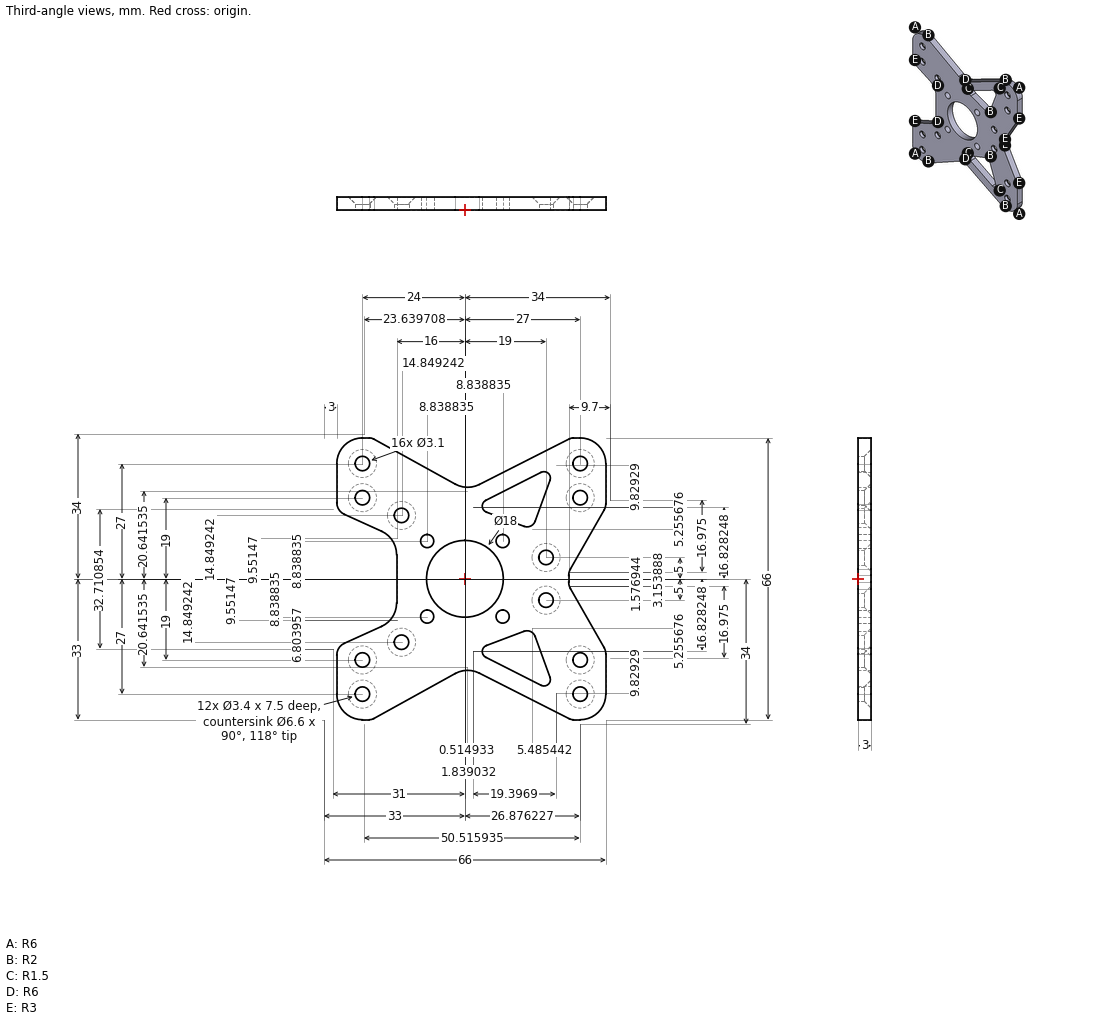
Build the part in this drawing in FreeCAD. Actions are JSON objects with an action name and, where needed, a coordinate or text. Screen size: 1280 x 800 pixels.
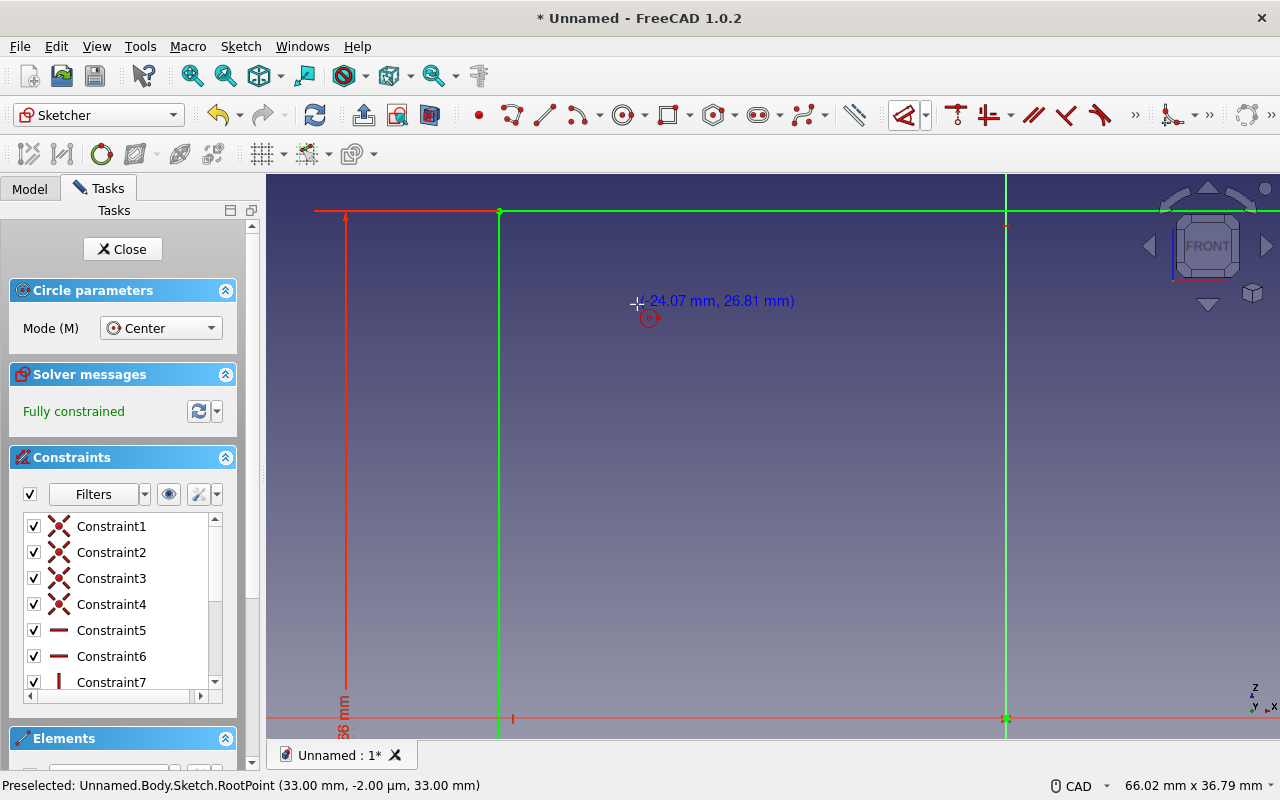
{"action": "left_click", "coordinate": [637, 303]}
{"action": "mouse_move", "coordinate": [654, 287]}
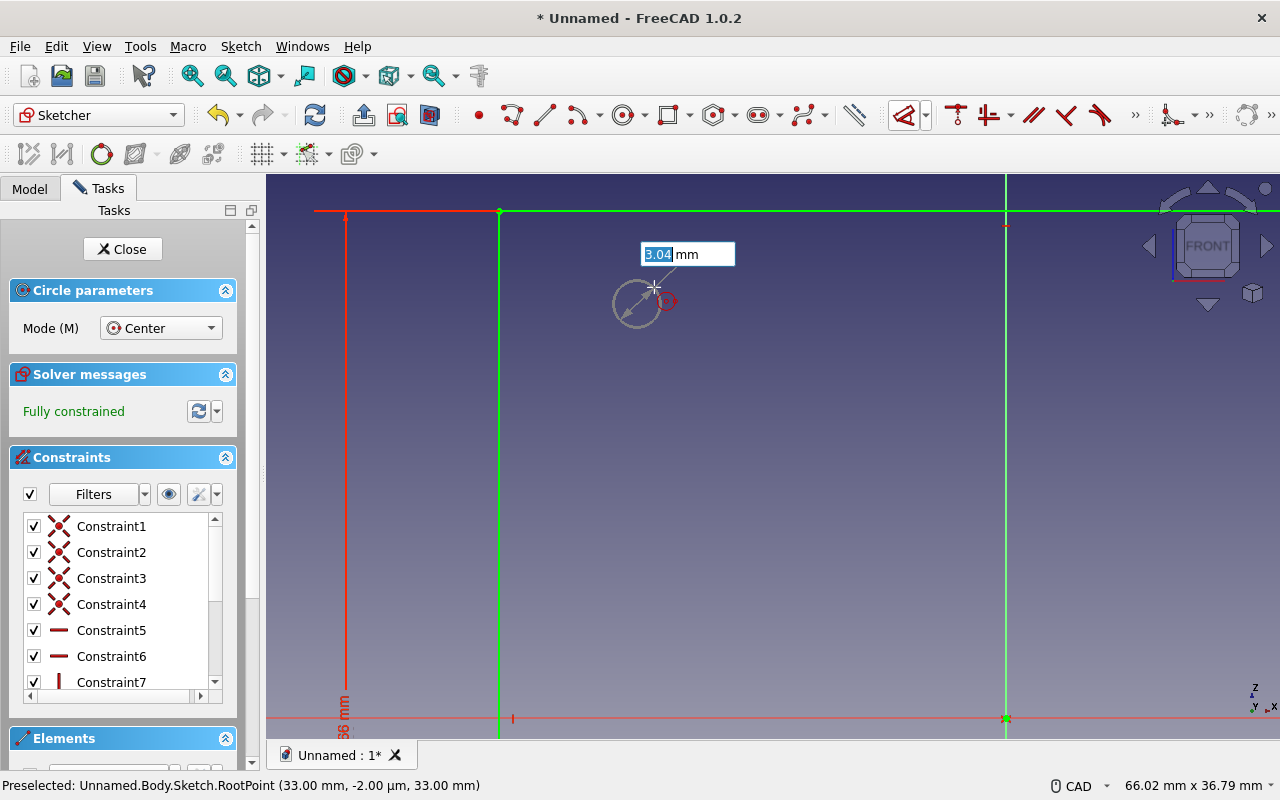
{"action": "type", "text": "3.1"}
{"action": "key", "text": "Return"}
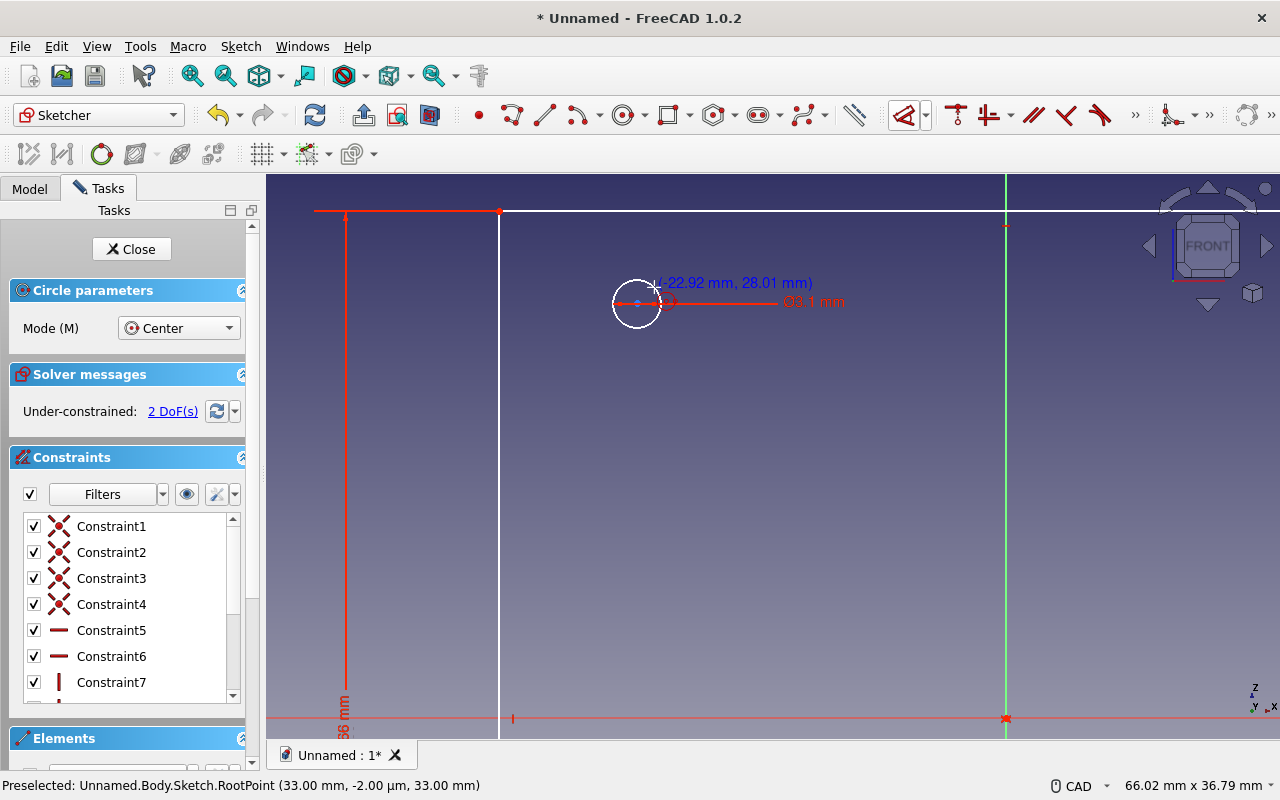
{"action": "left_click", "coordinate": [637, 426]}
{"action": "mouse_move", "coordinate": [654, 410]}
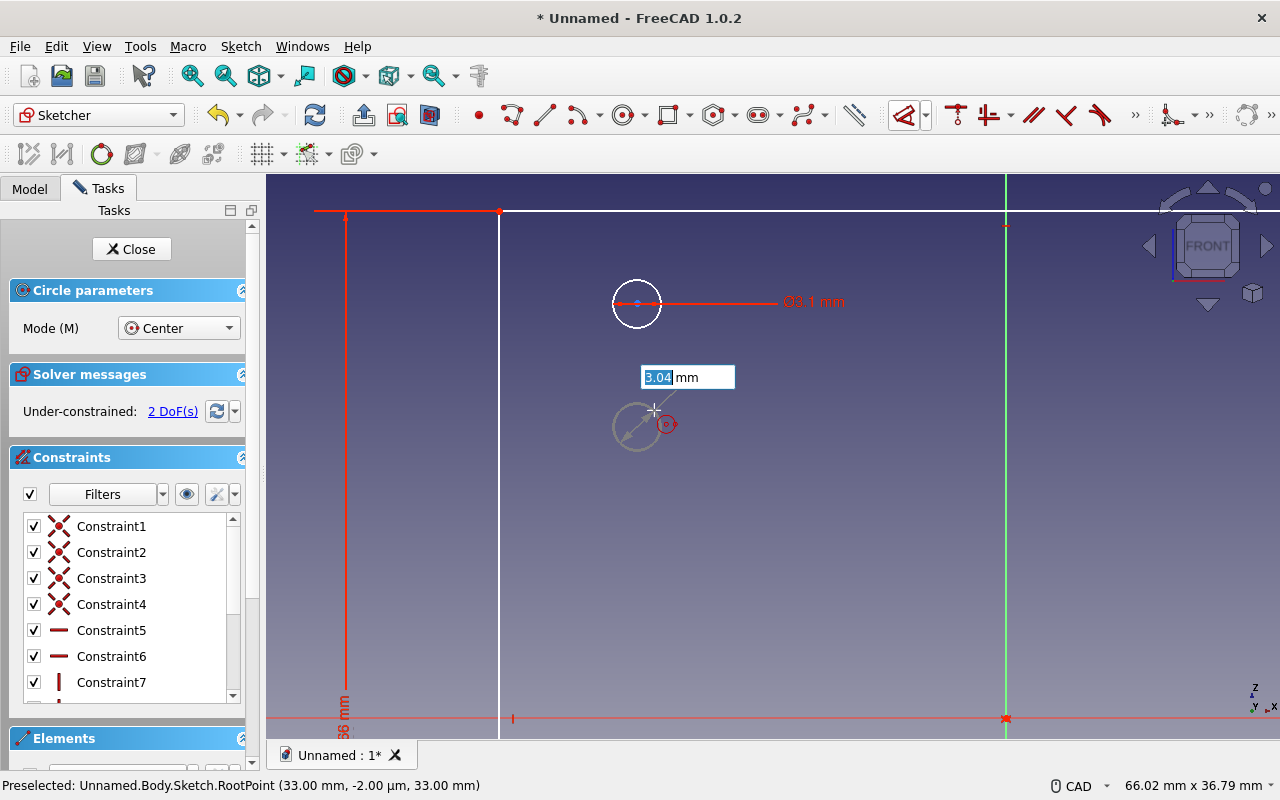
{"action": "type", "text": "3.1"}
{"action": "key", "text": "Return"}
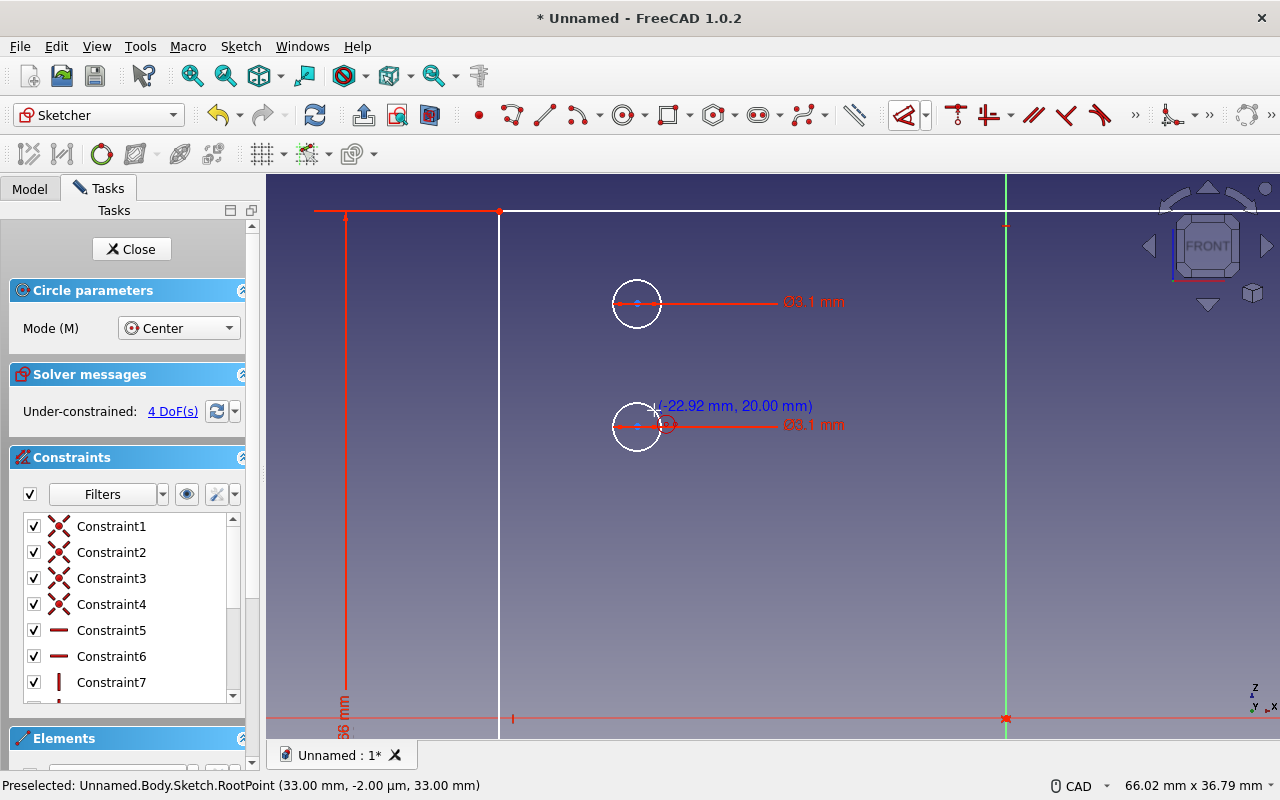
{"action": "left_click", "coordinate": [778, 490]}
{"action": "mouse_move", "coordinate": [795, 473]}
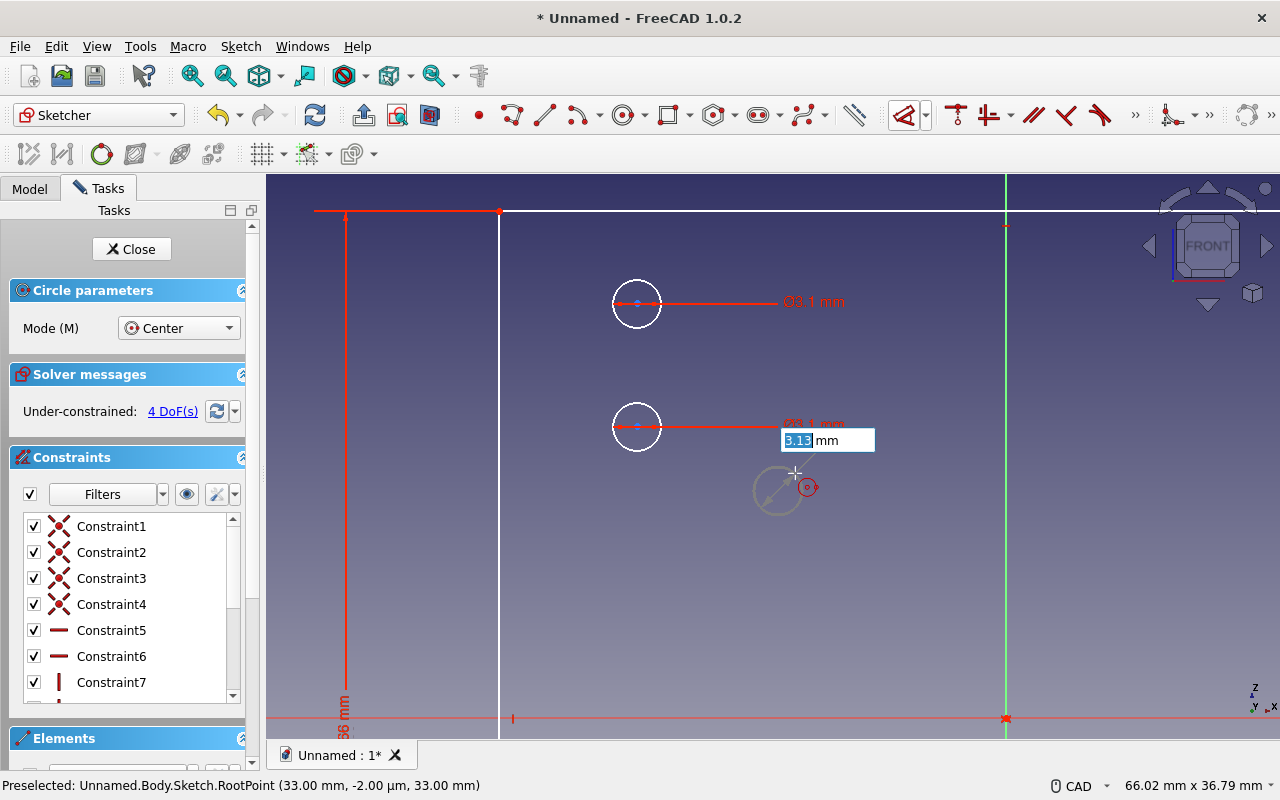
{"action": "type", "text": "3.1"}
{"action": "key", "text": "Return"}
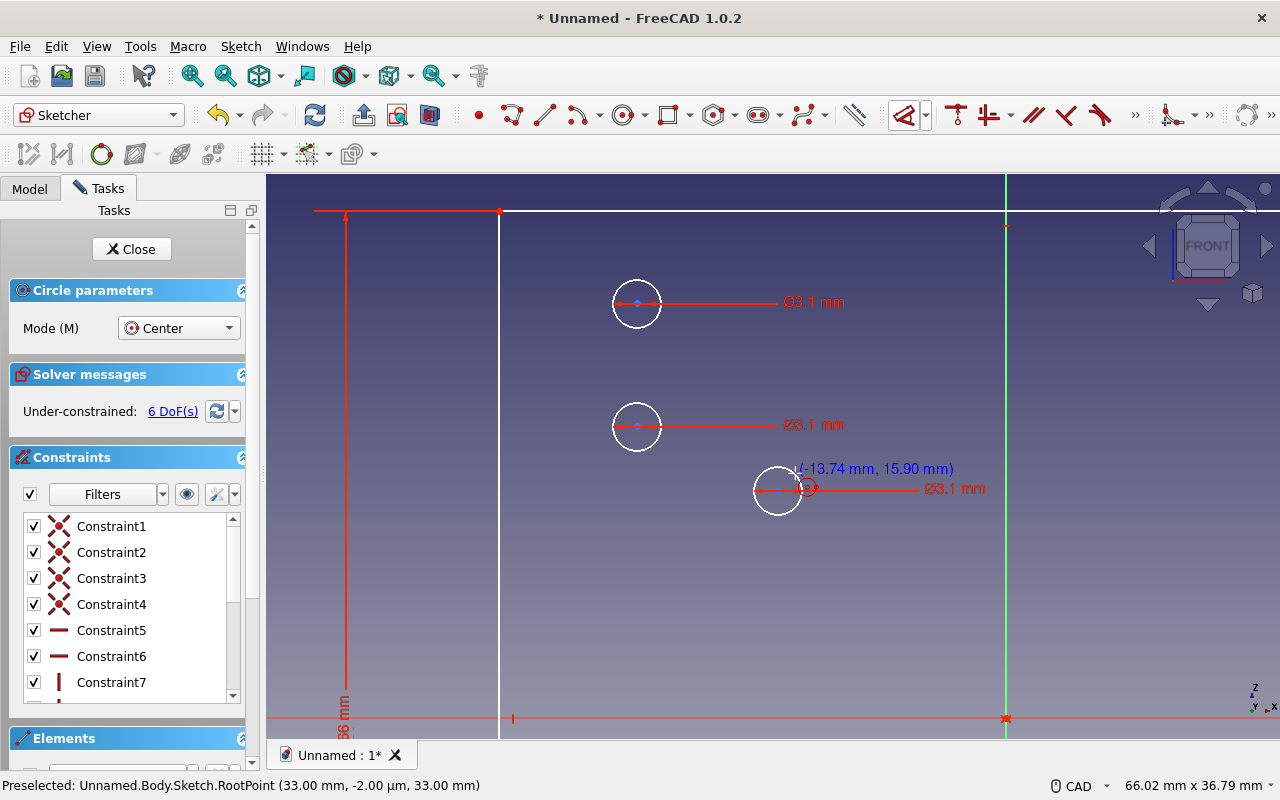
{"action": "left_click", "coordinate": [870, 582]}
{"action": "mouse_move", "coordinate": [887, 566]}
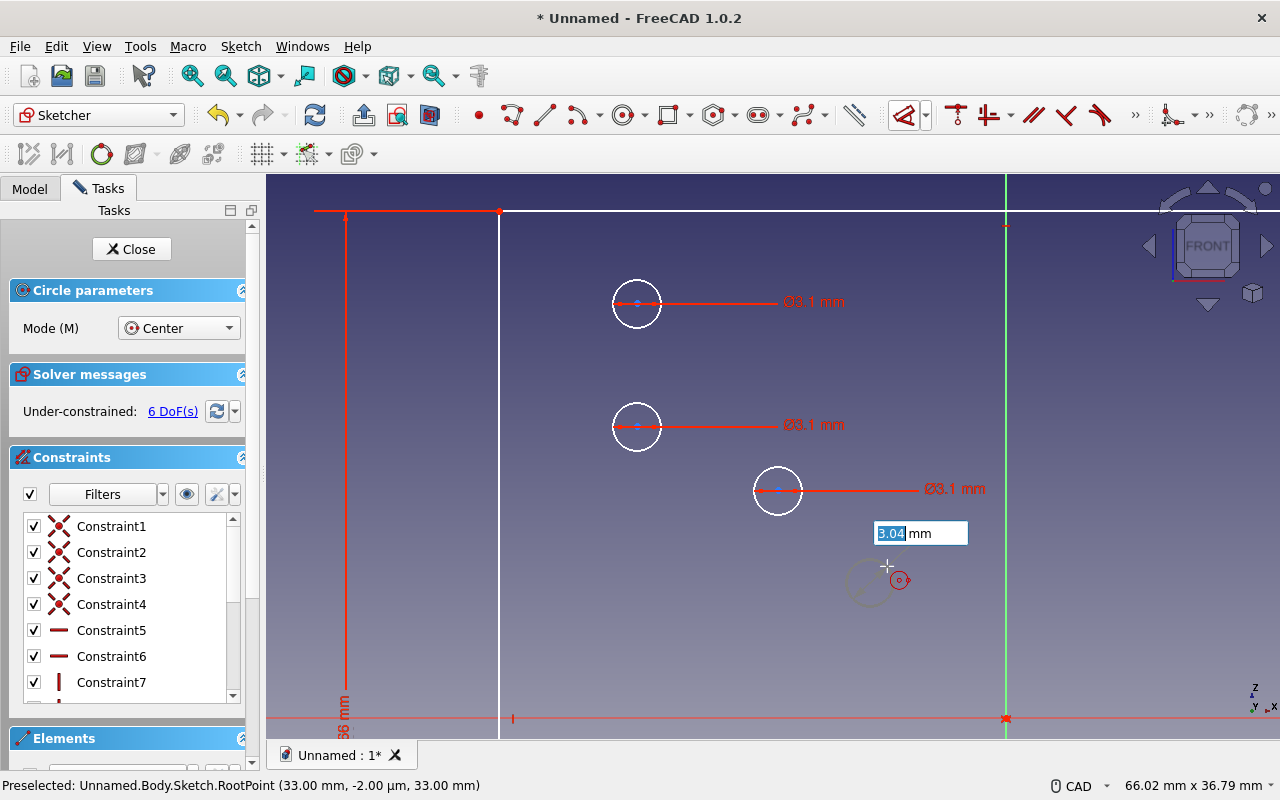
{"action": "type", "text": "3.1"}
{"action": "key", "text": "Return"}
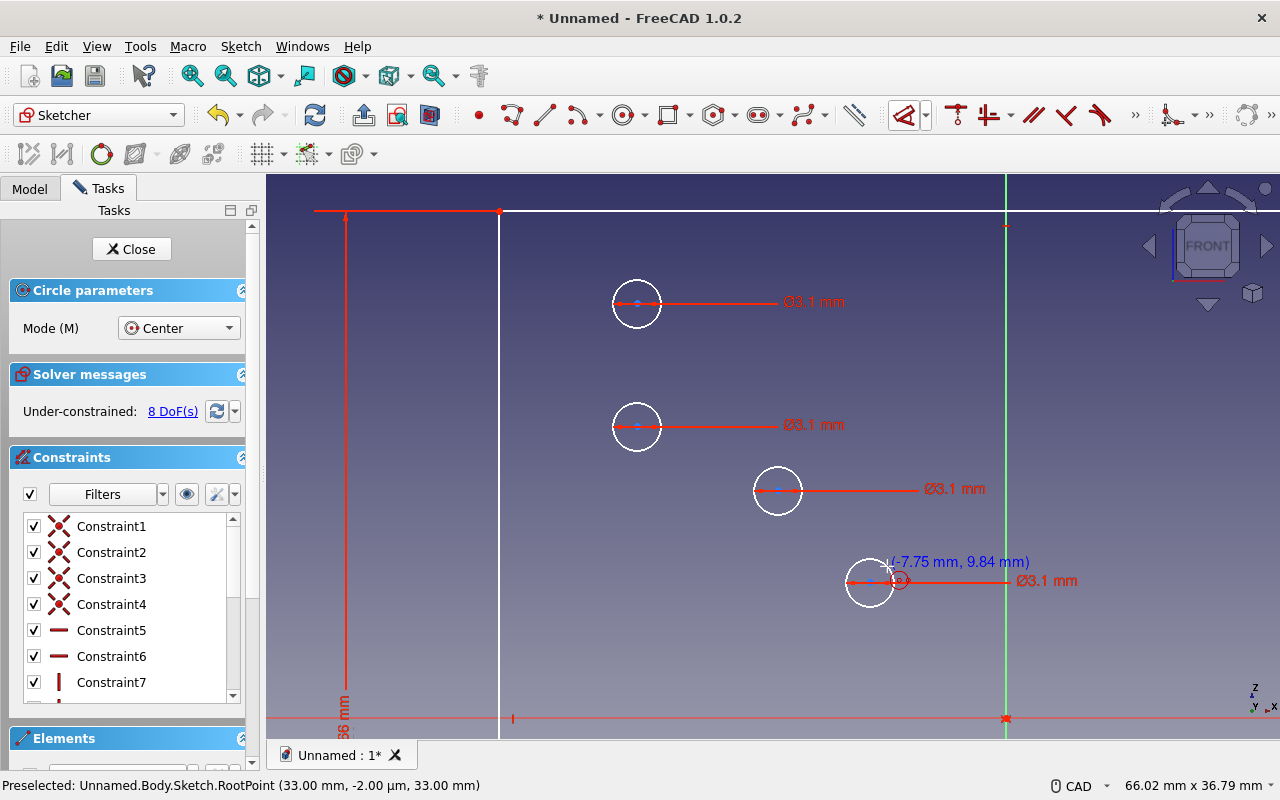
{"action": "scroll", "coordinate": [529, 304], "scroll_direction": "down", "scroll_amount": 5}